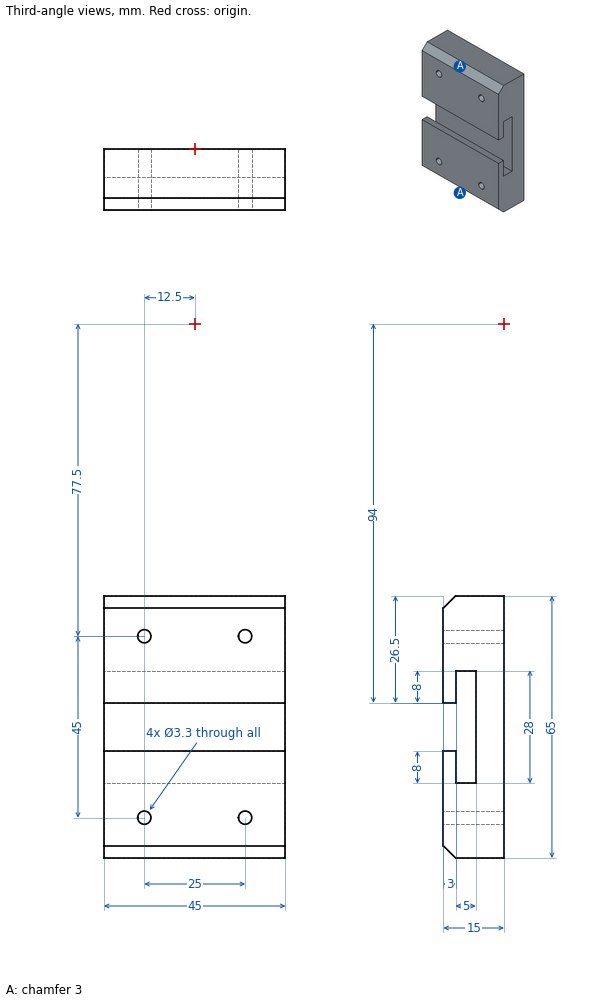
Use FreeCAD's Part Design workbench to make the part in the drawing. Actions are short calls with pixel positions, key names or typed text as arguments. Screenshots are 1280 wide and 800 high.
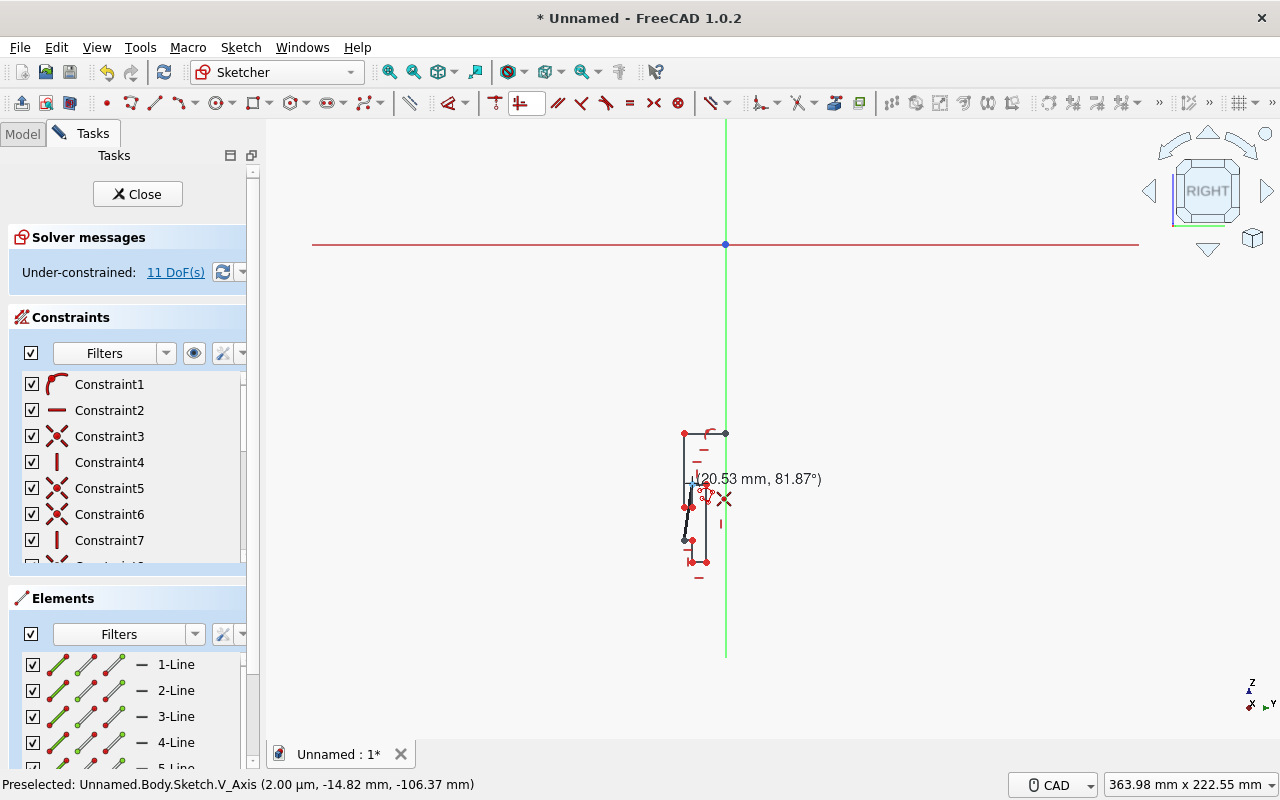
click(684, 614)
click(717, 614)
click(726, 434)
key(Escape)
key(Escape)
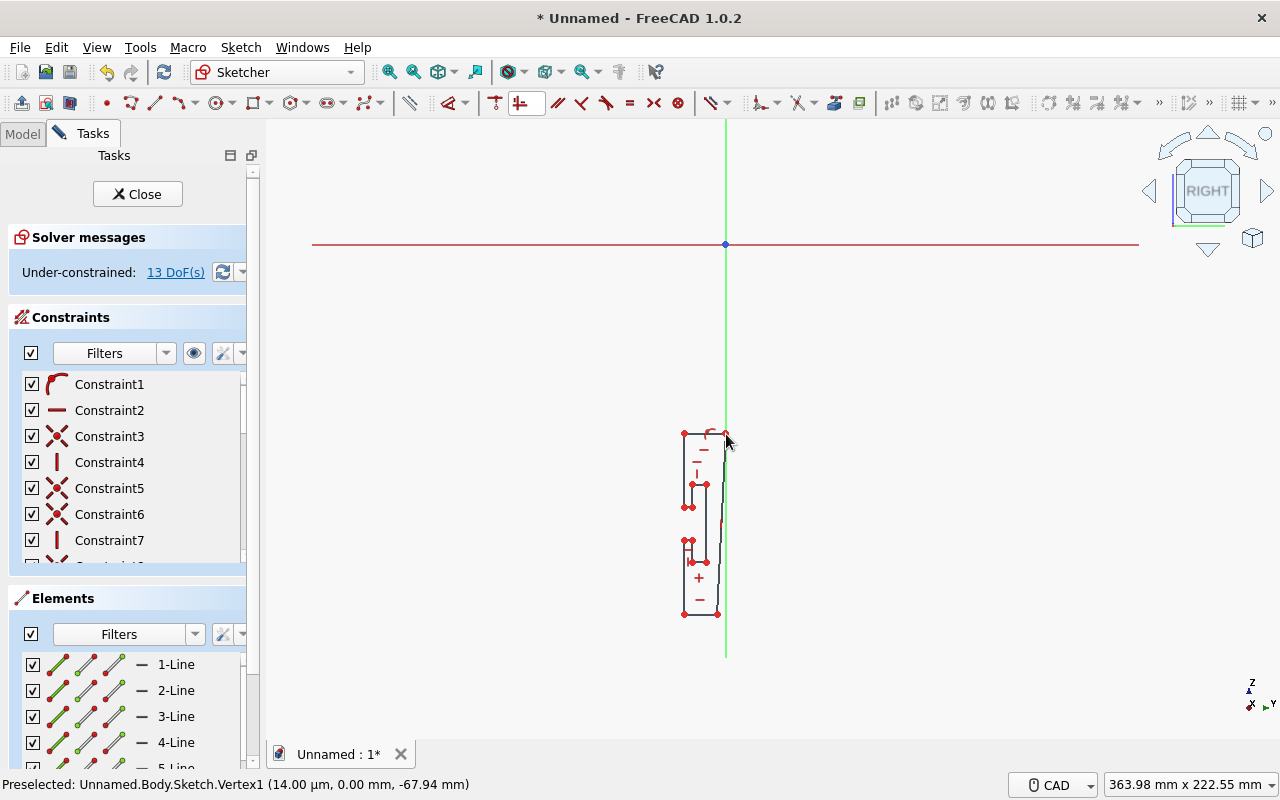
scroll(688, 507, up, 7)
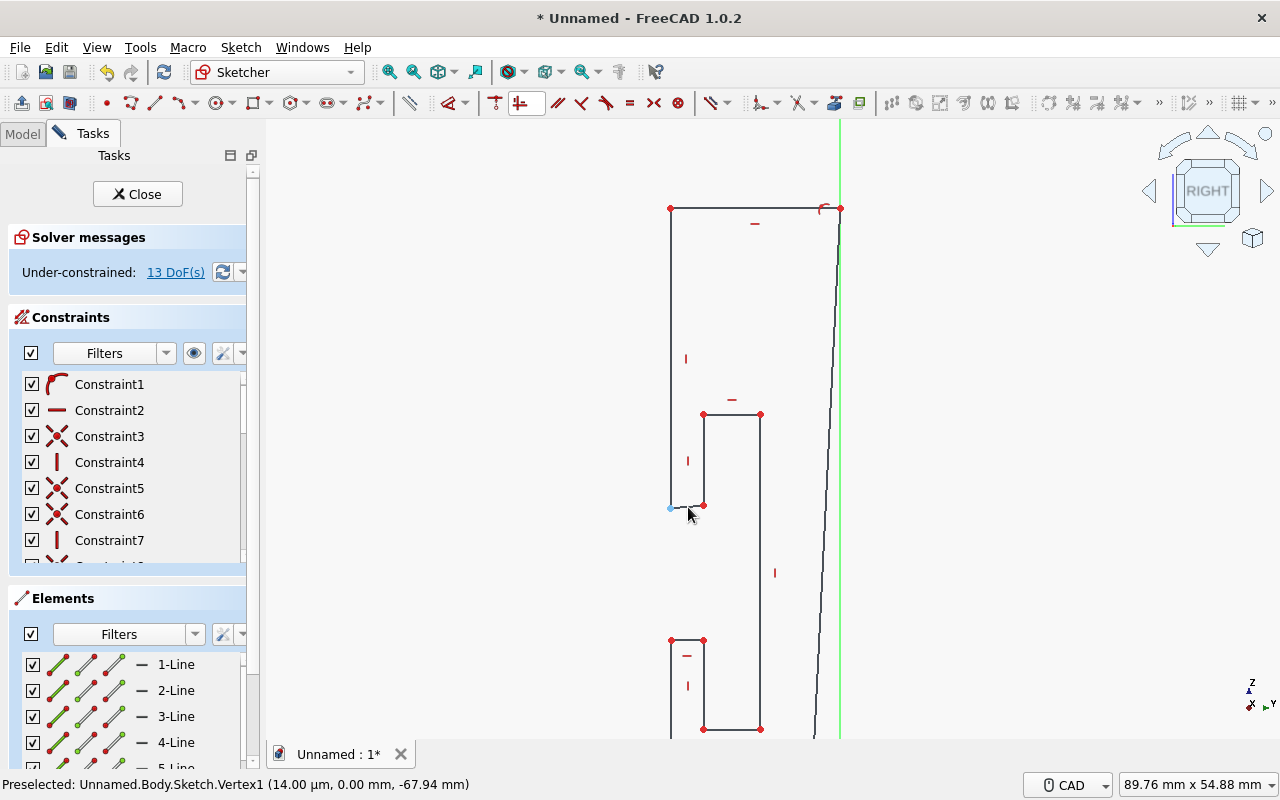
click(687, 507)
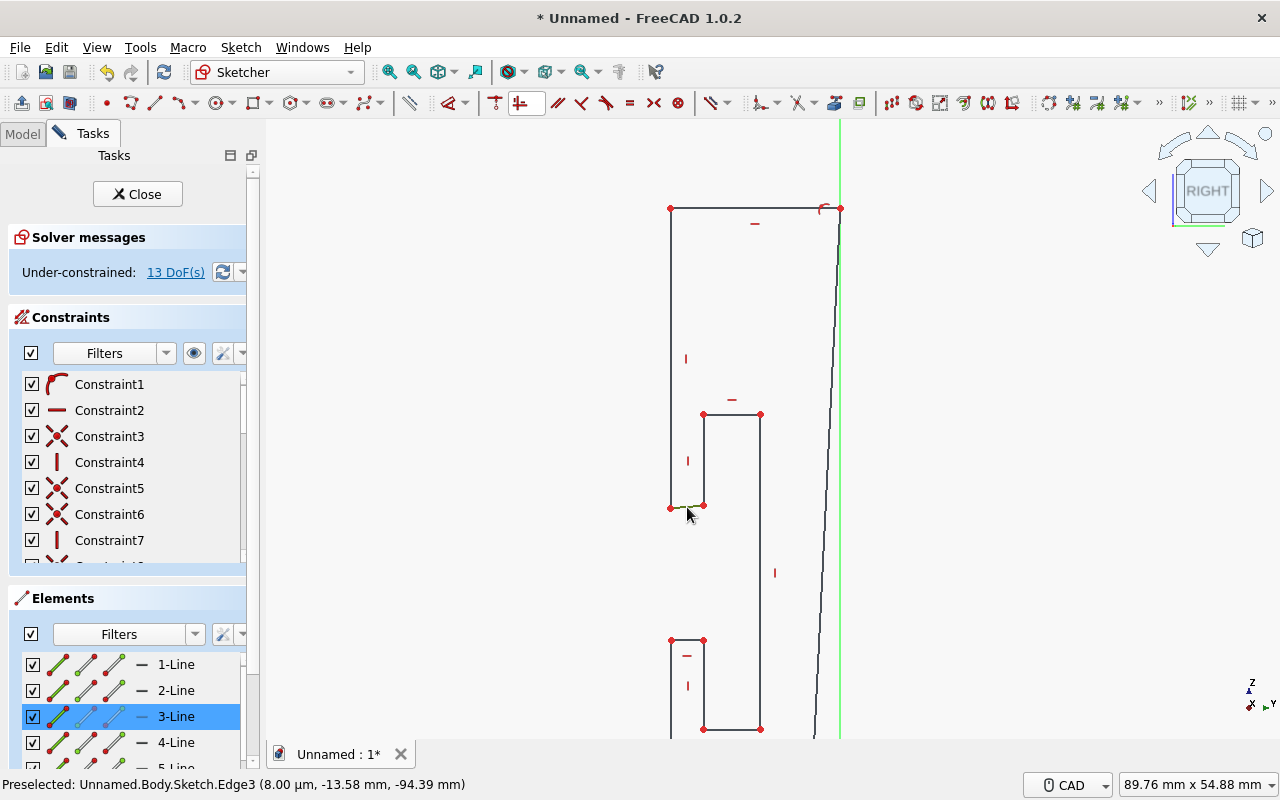
click(540, 104)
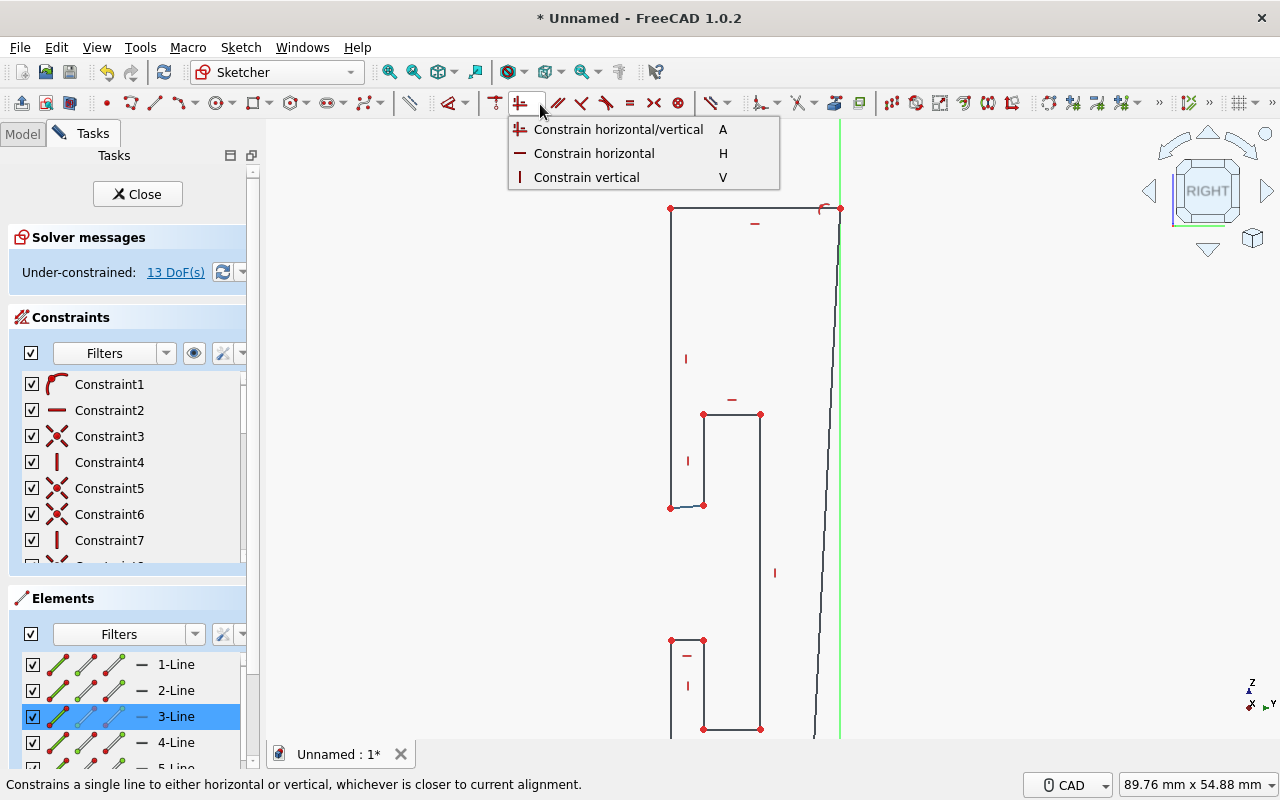
click(644, 153)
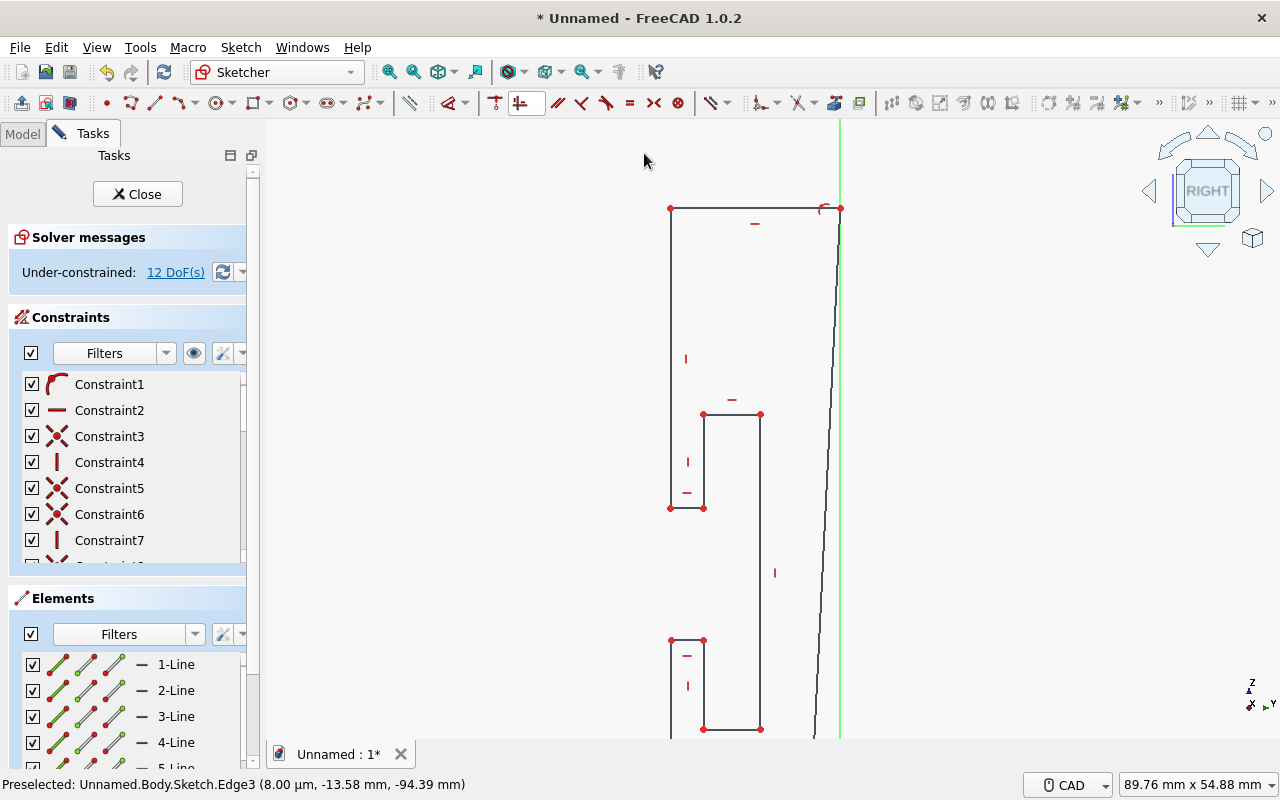
scroll(830, 429, up, 2)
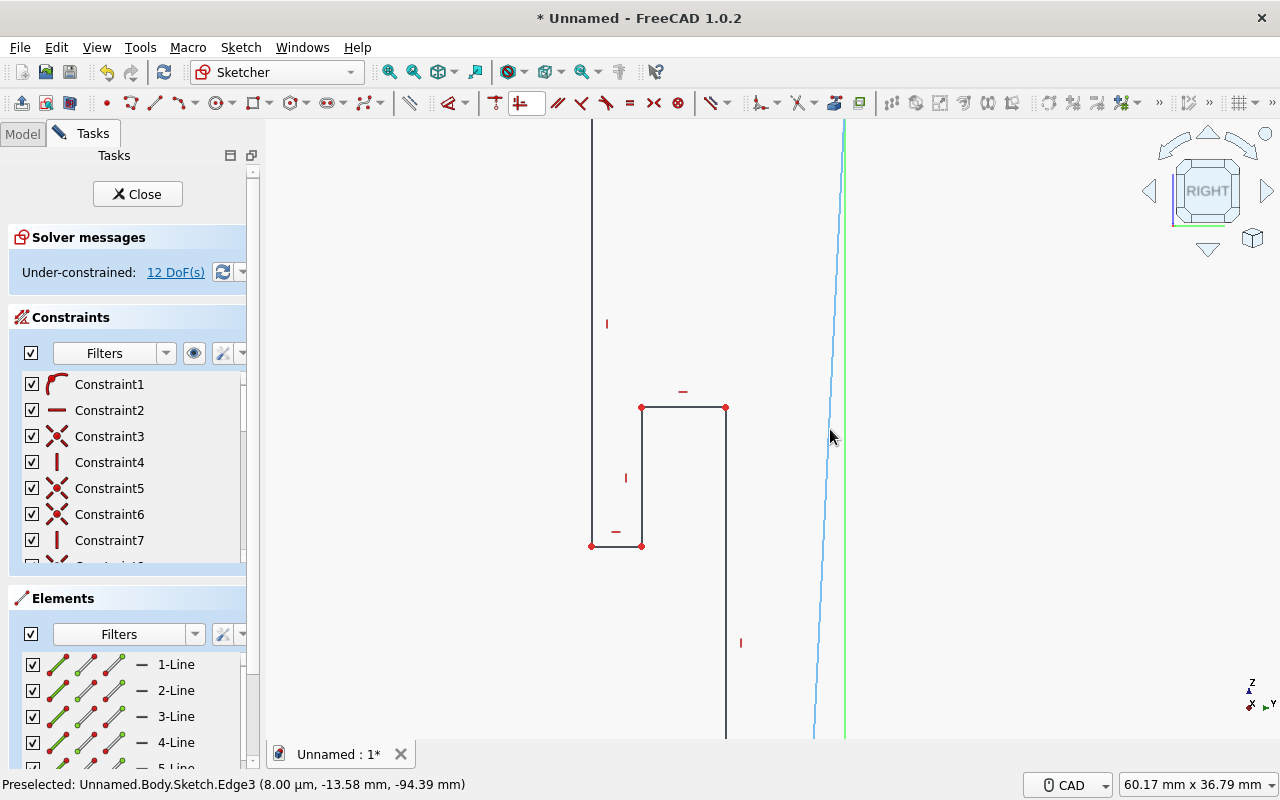
click(829, 428)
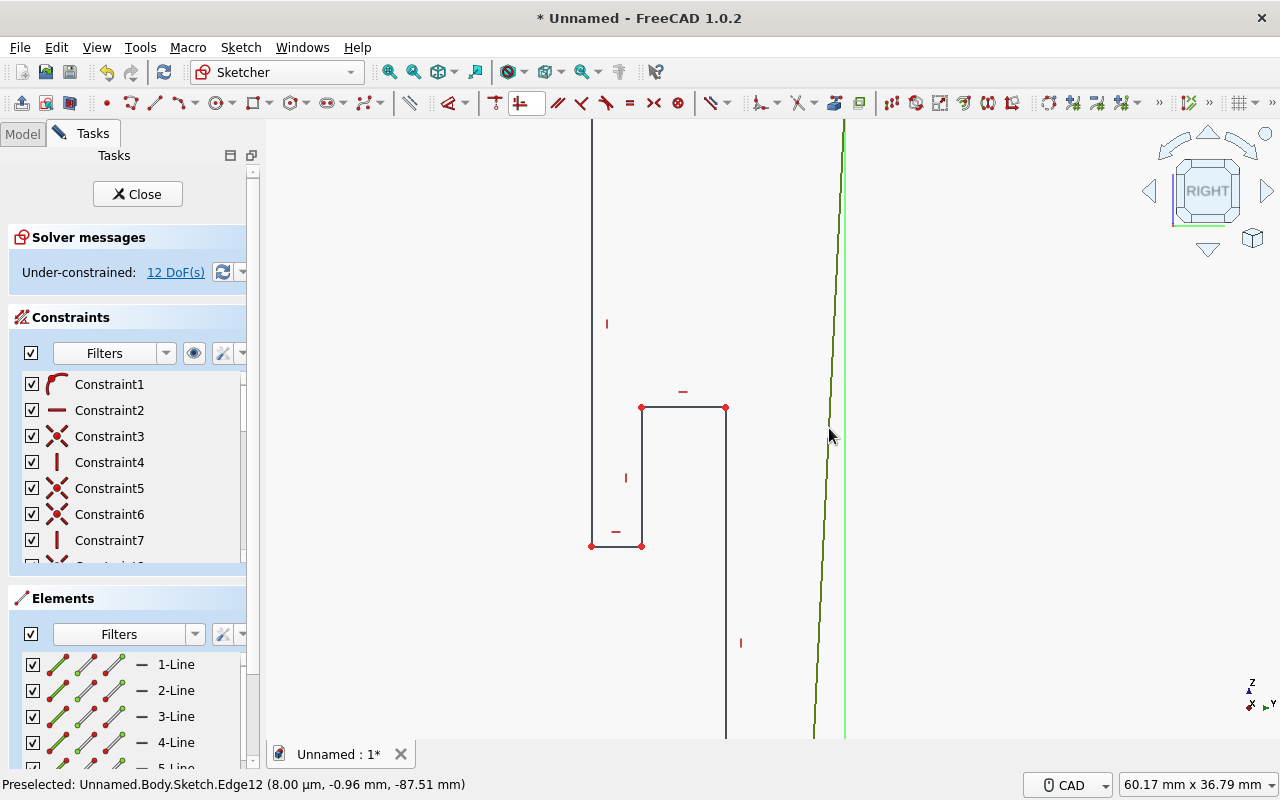
click(540, 104)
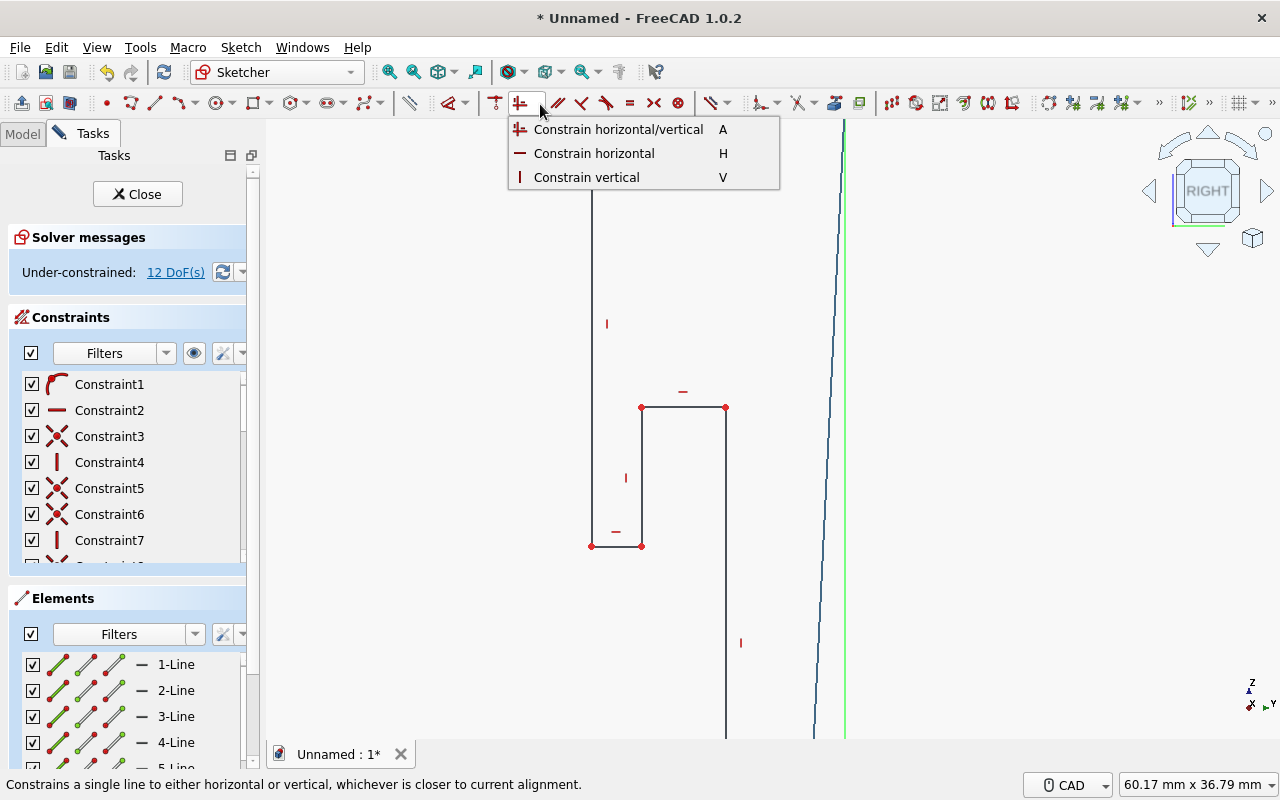
click(644, 177)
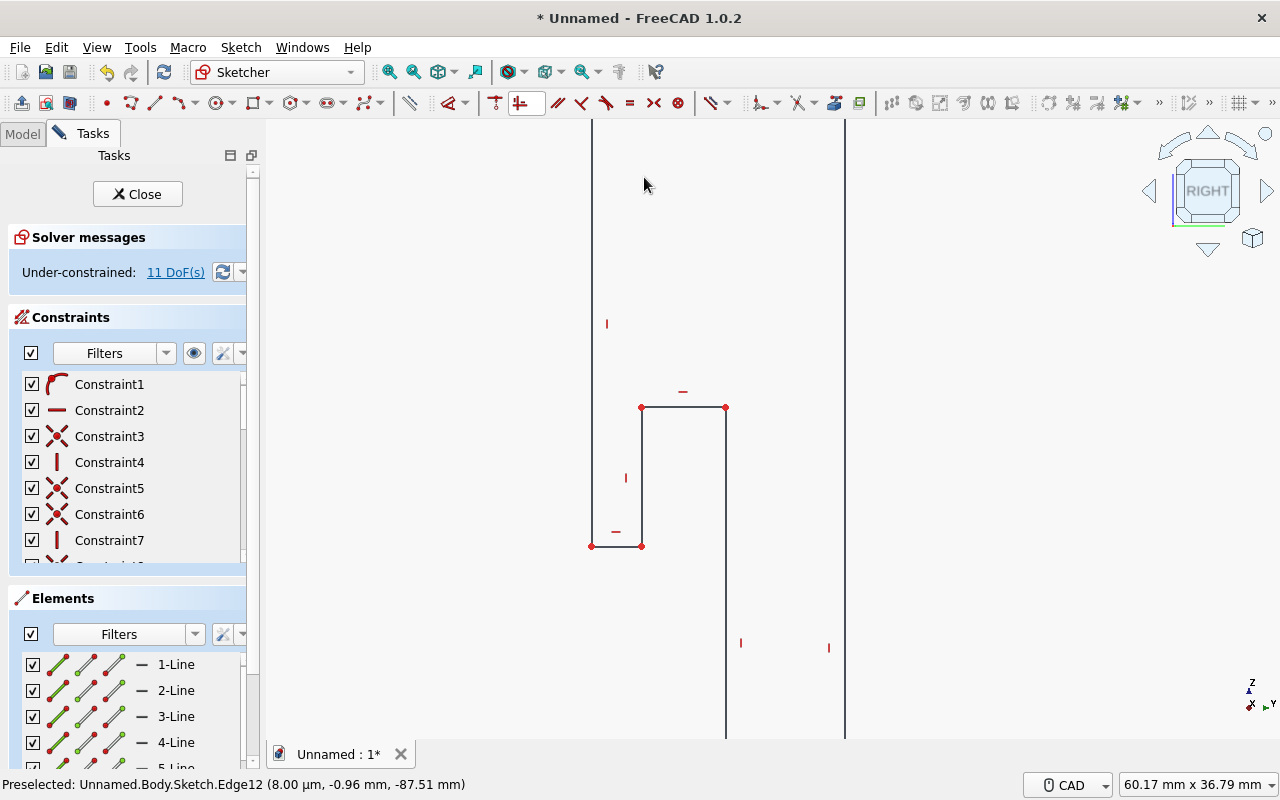
click(607, 547)